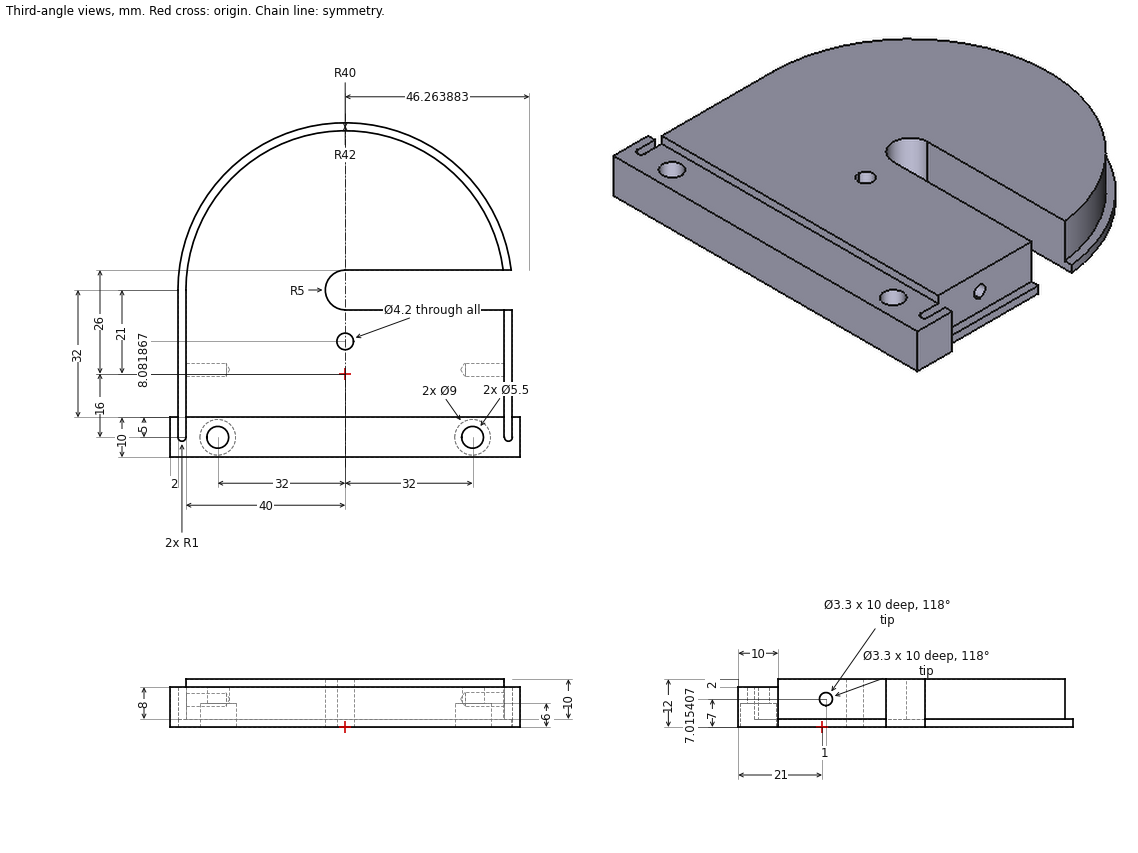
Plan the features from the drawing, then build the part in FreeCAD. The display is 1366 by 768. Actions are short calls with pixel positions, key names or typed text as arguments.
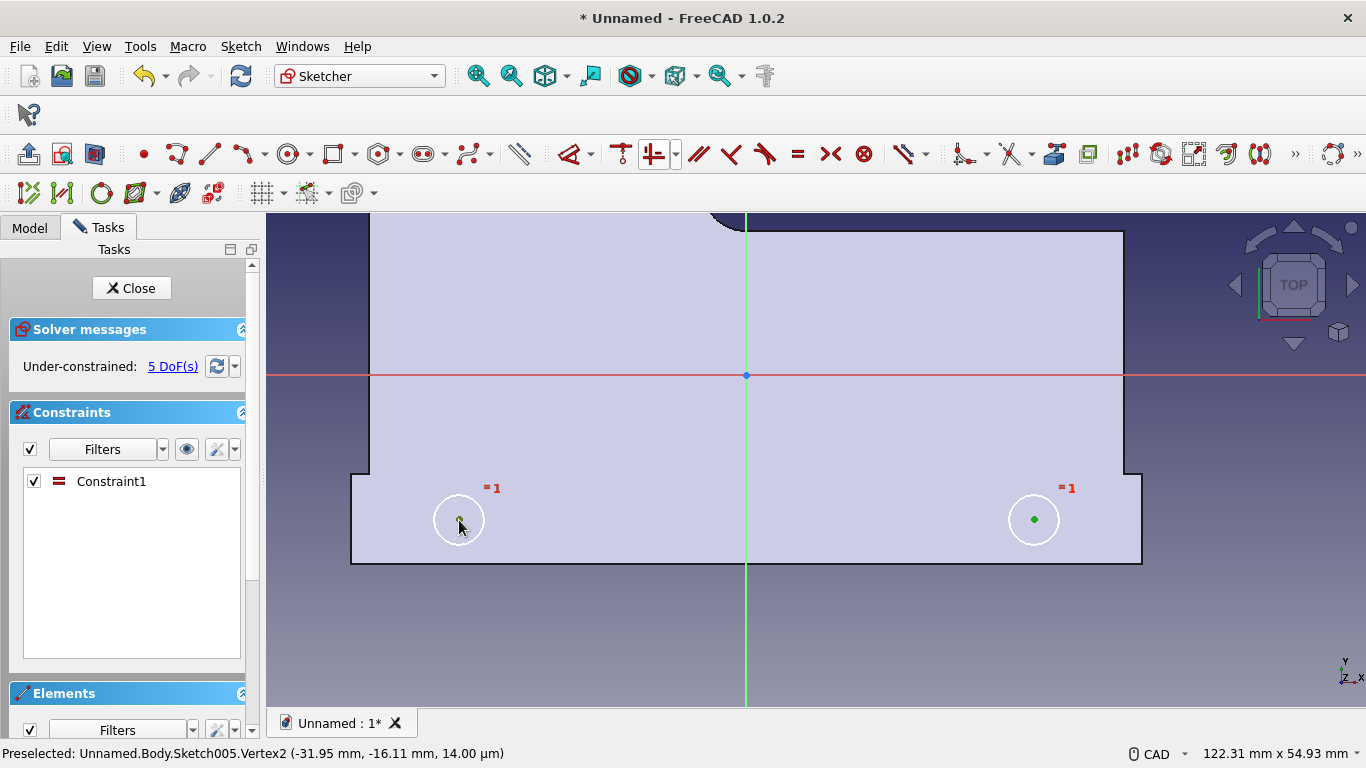
key(h)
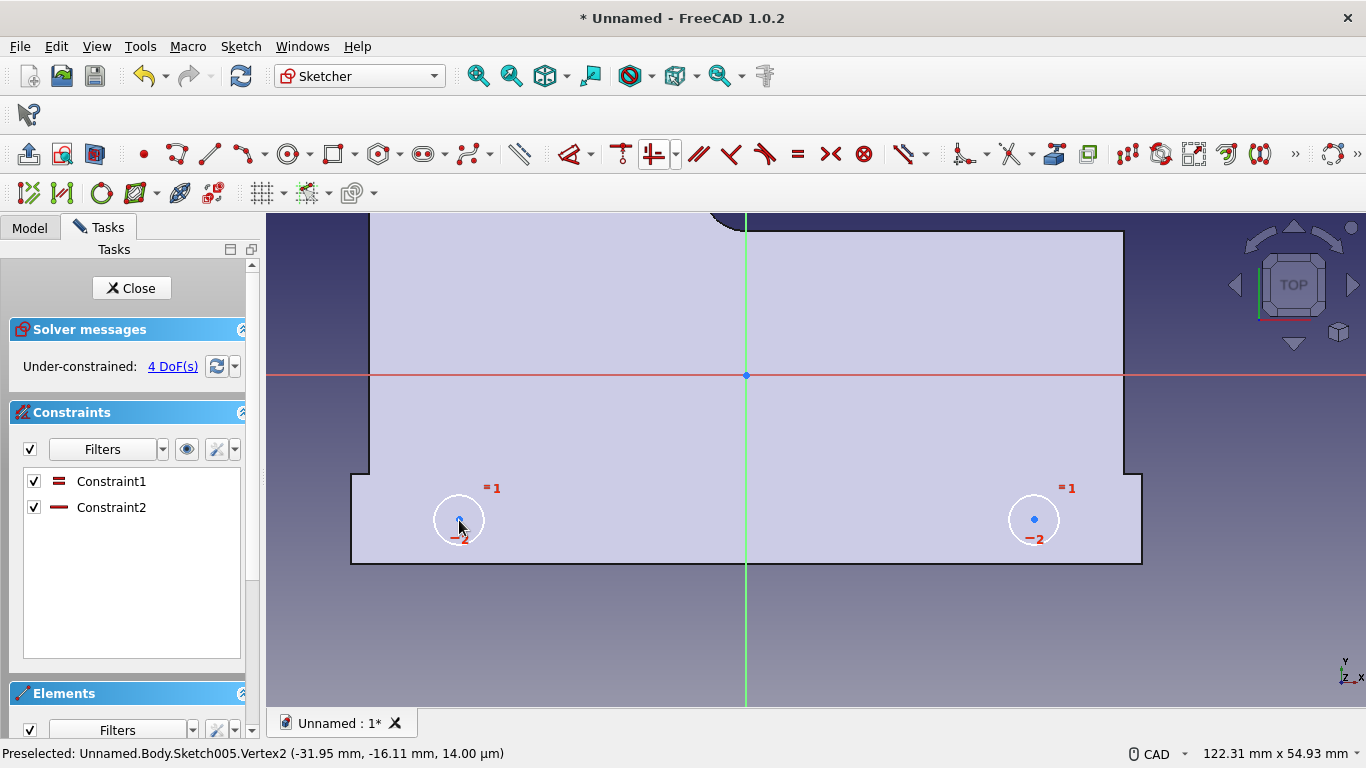
key(d)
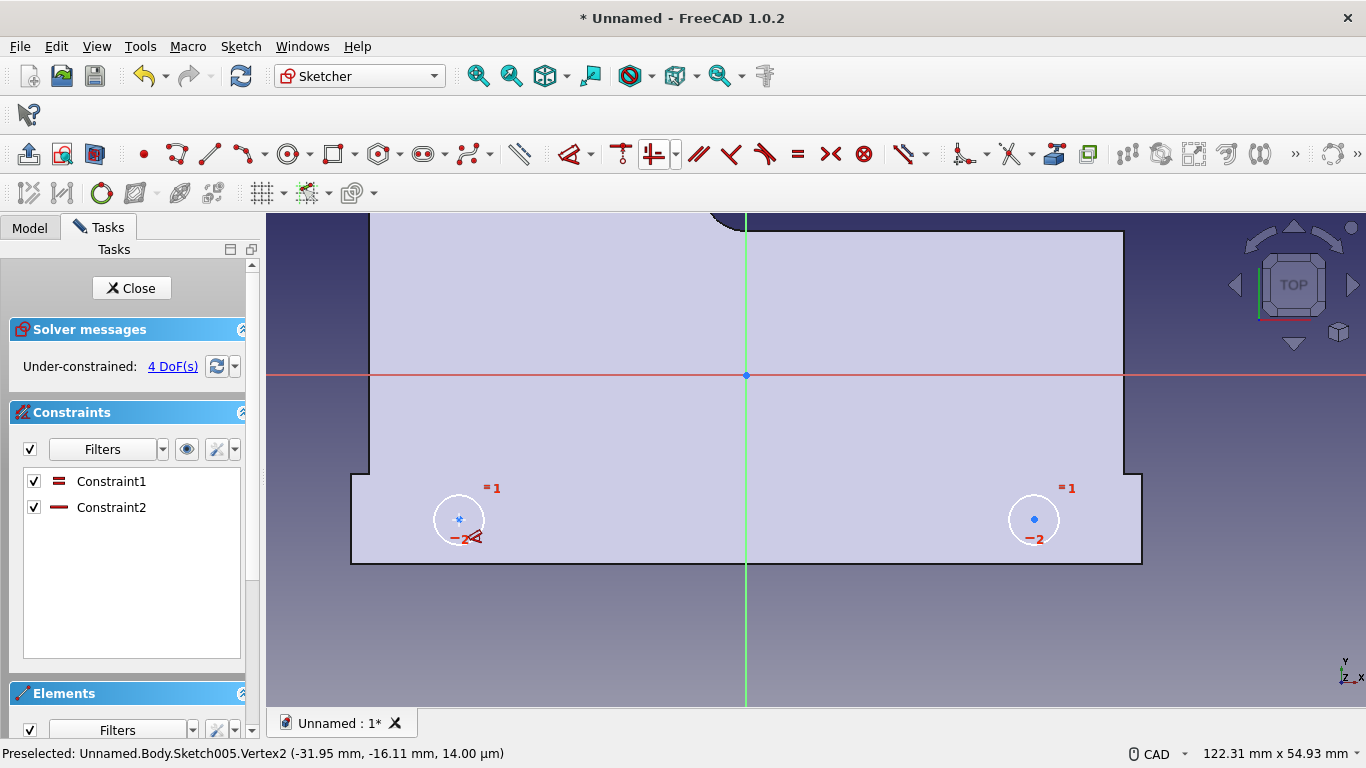
click(1051, 502)
click(1073, 479)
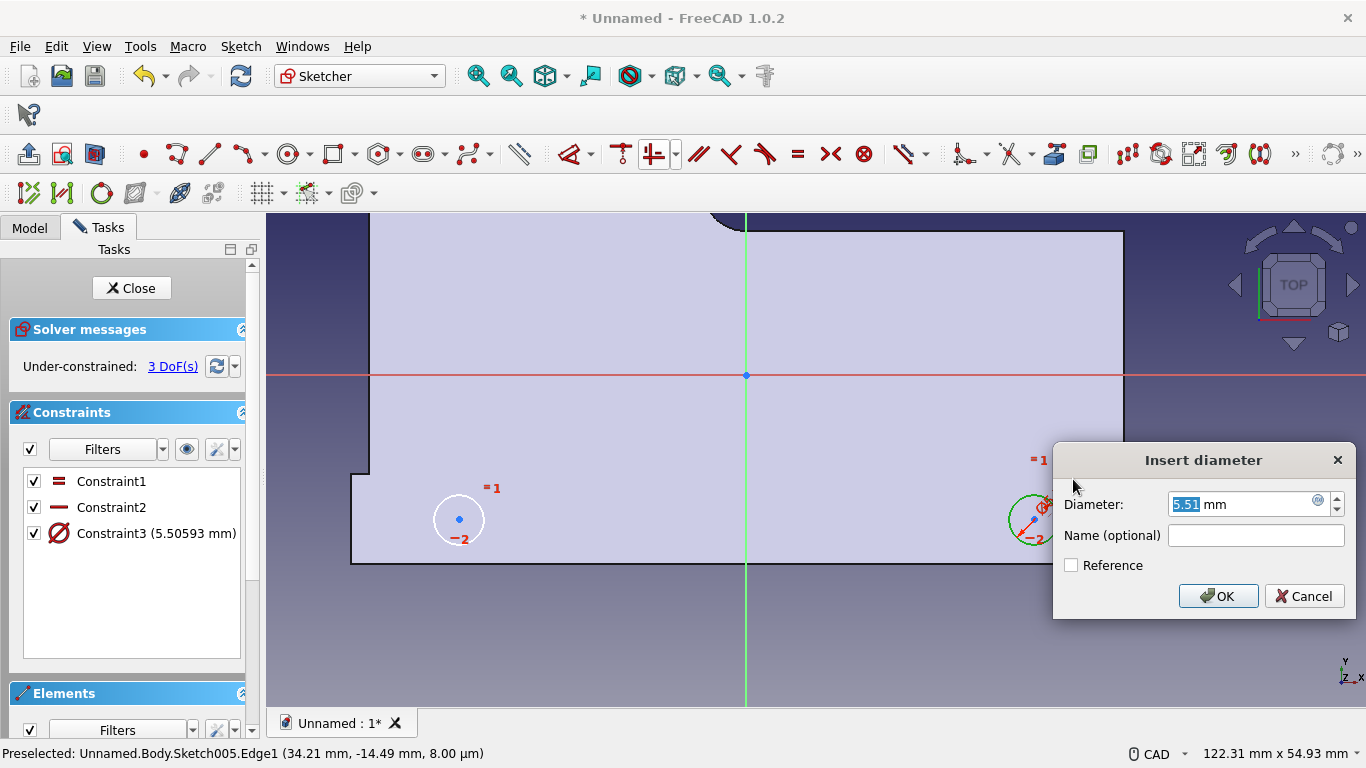
text(5.5)
key(Return)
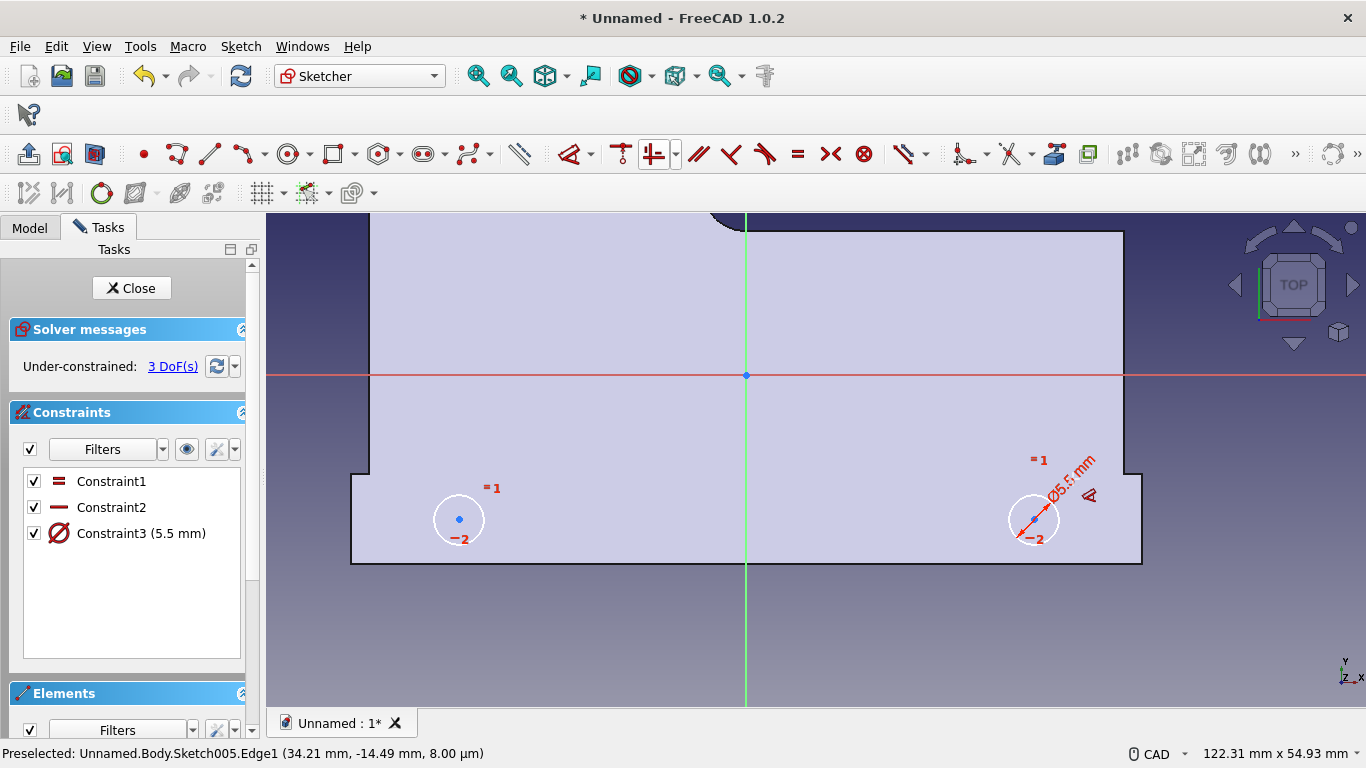
click(1034, 520)
click(890, 341)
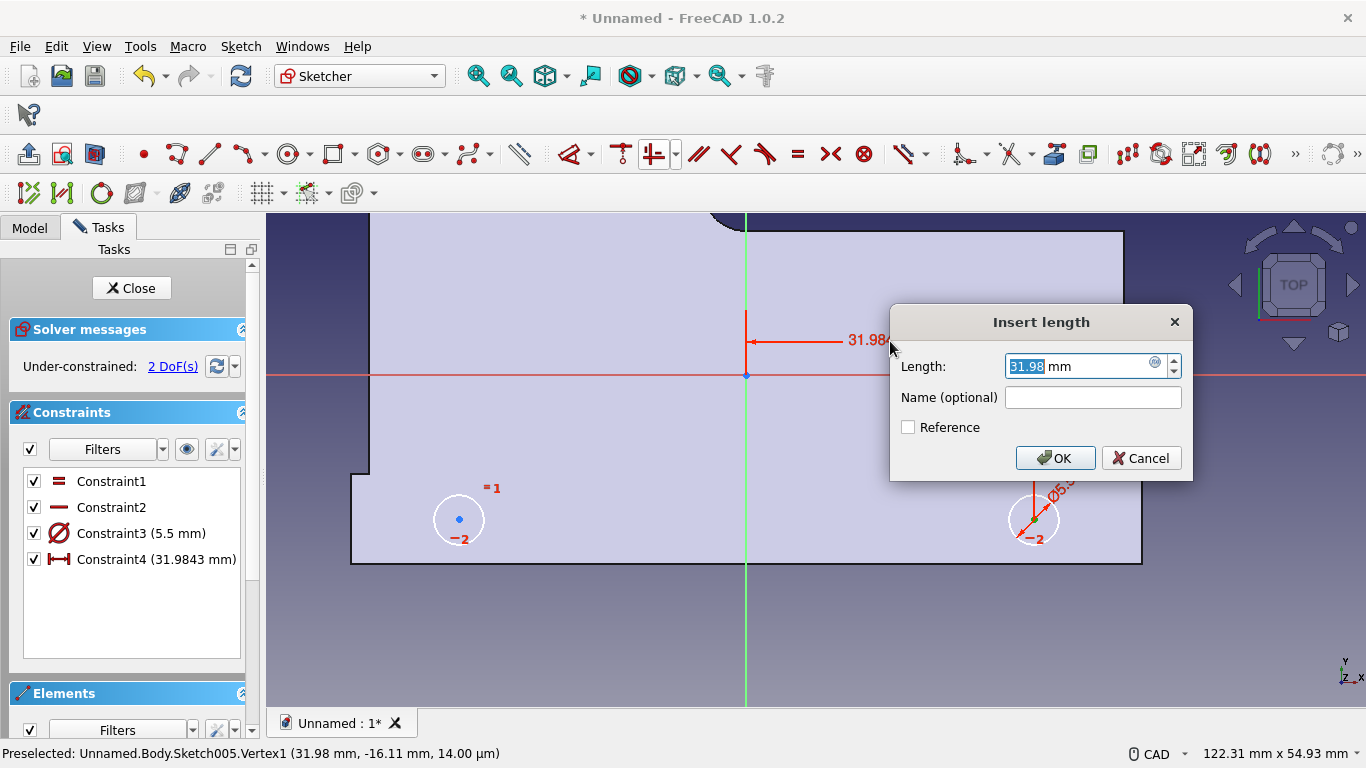
text(32)
key(Return)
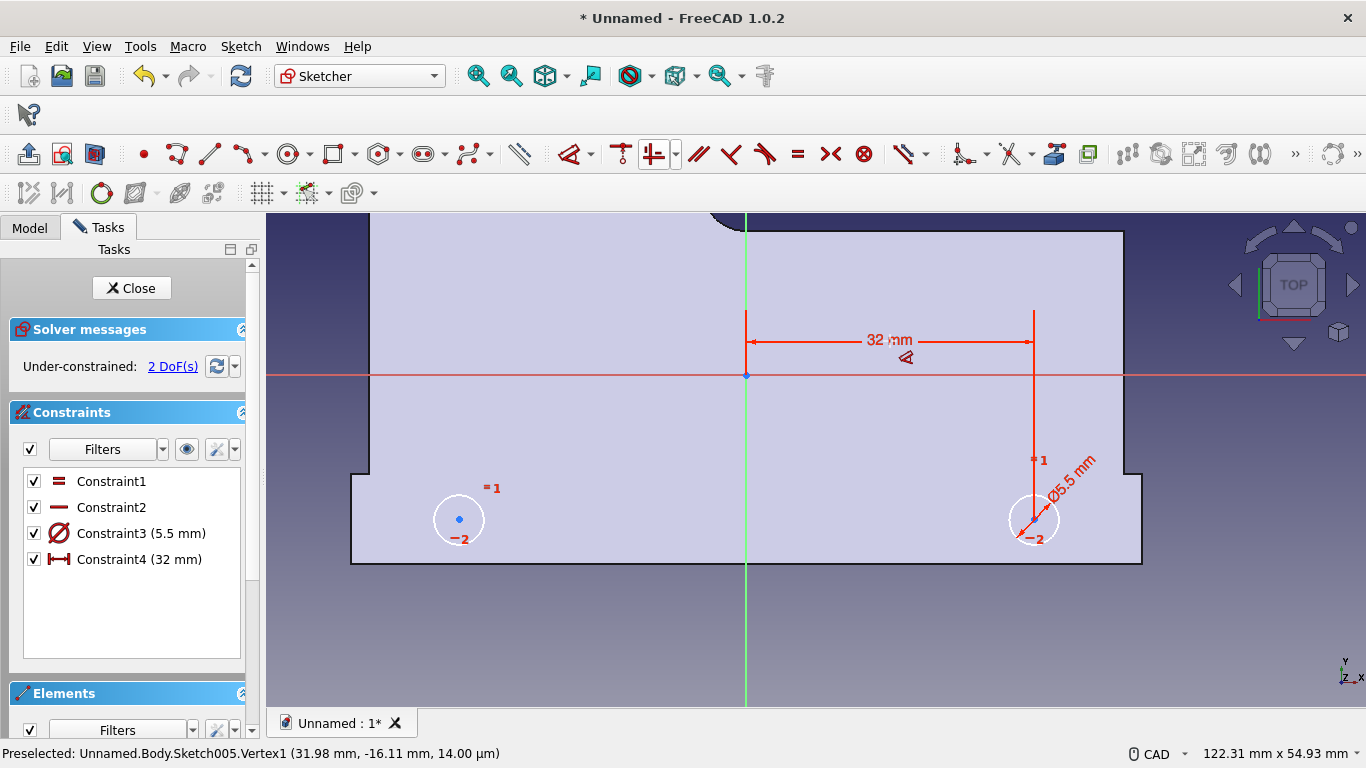
click(1034, 520)
click(1068, 448)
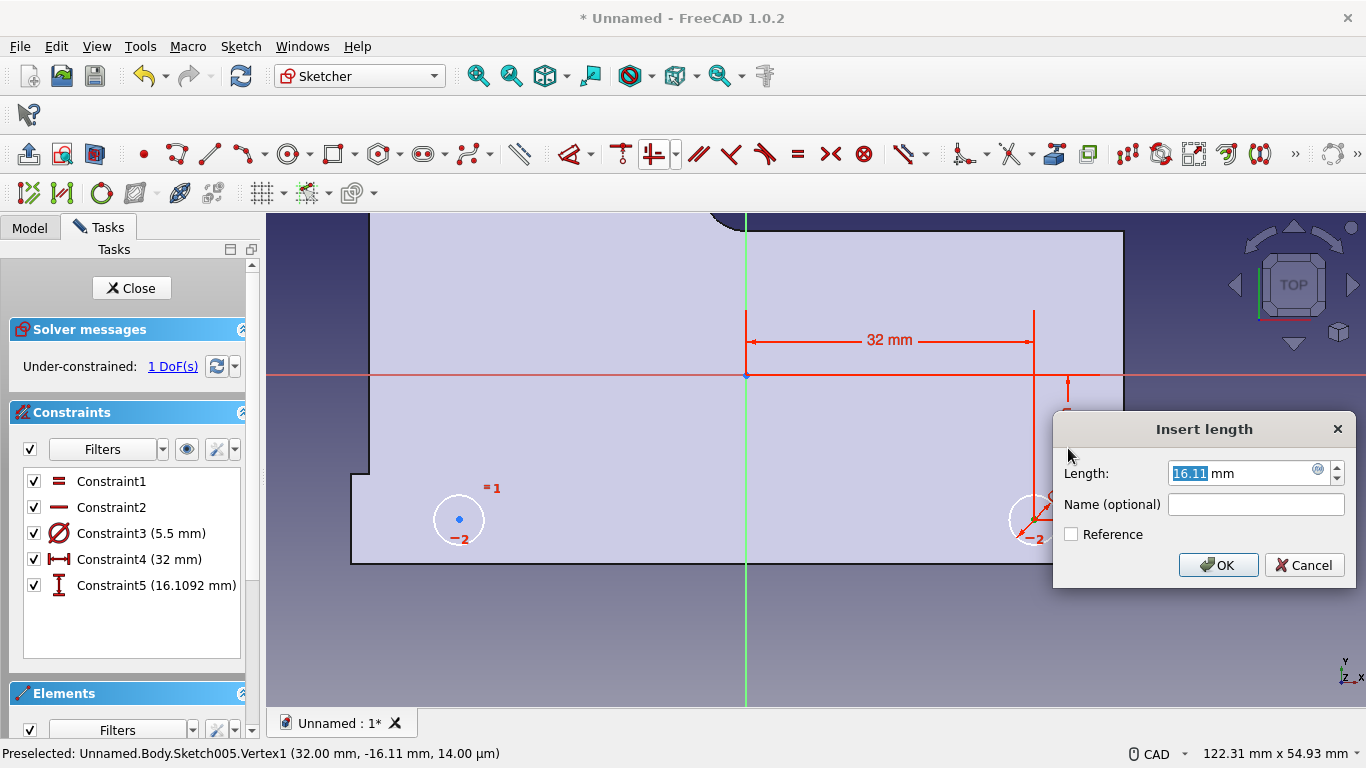
text(16)
key(Return)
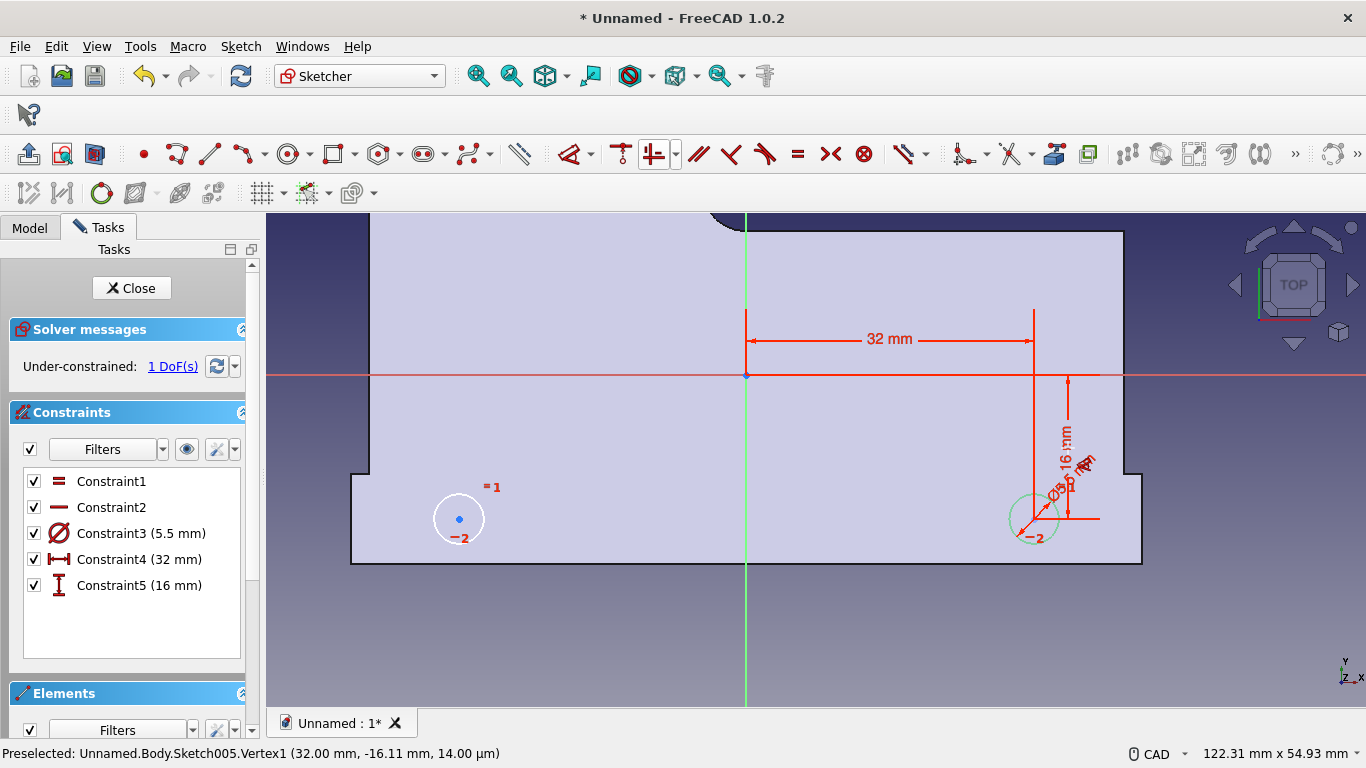
click(459, 519)
click(603, 341)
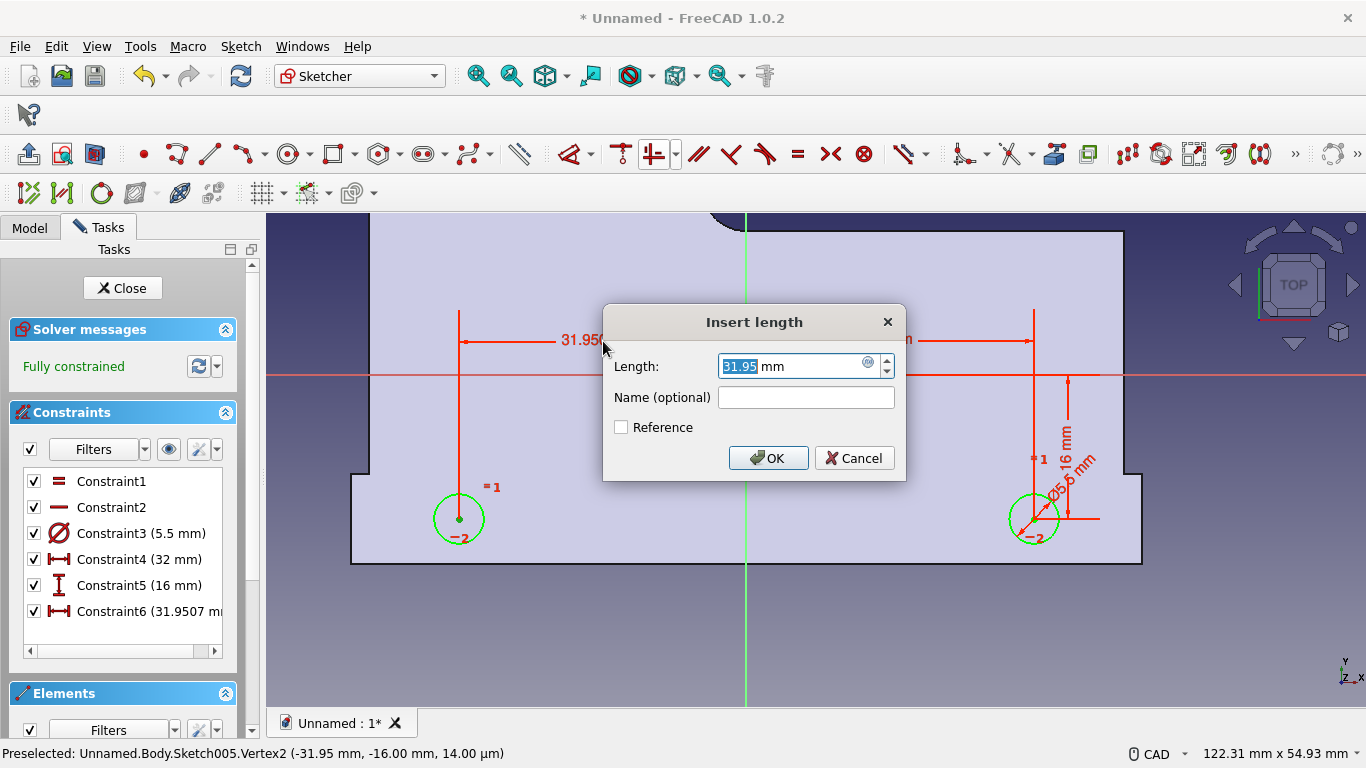
text(32)
key(Return)
key(Escape)